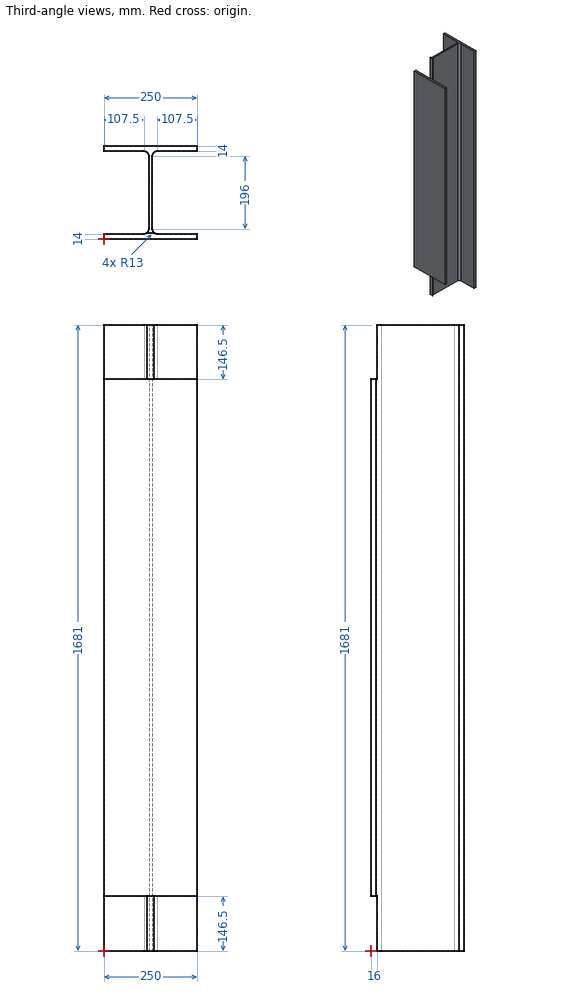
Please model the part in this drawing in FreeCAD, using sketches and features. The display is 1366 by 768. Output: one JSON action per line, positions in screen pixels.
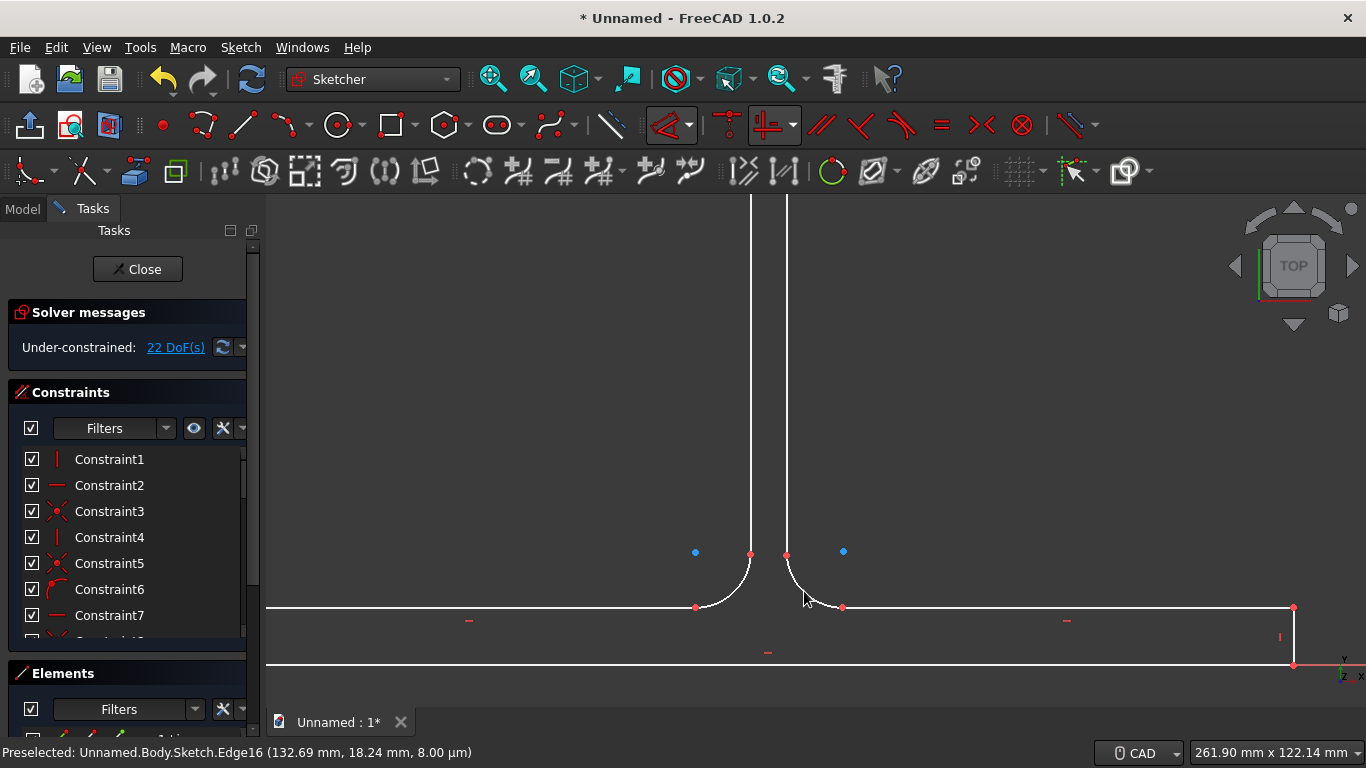
{"action": "left_click", "coordinate": [787, 309]}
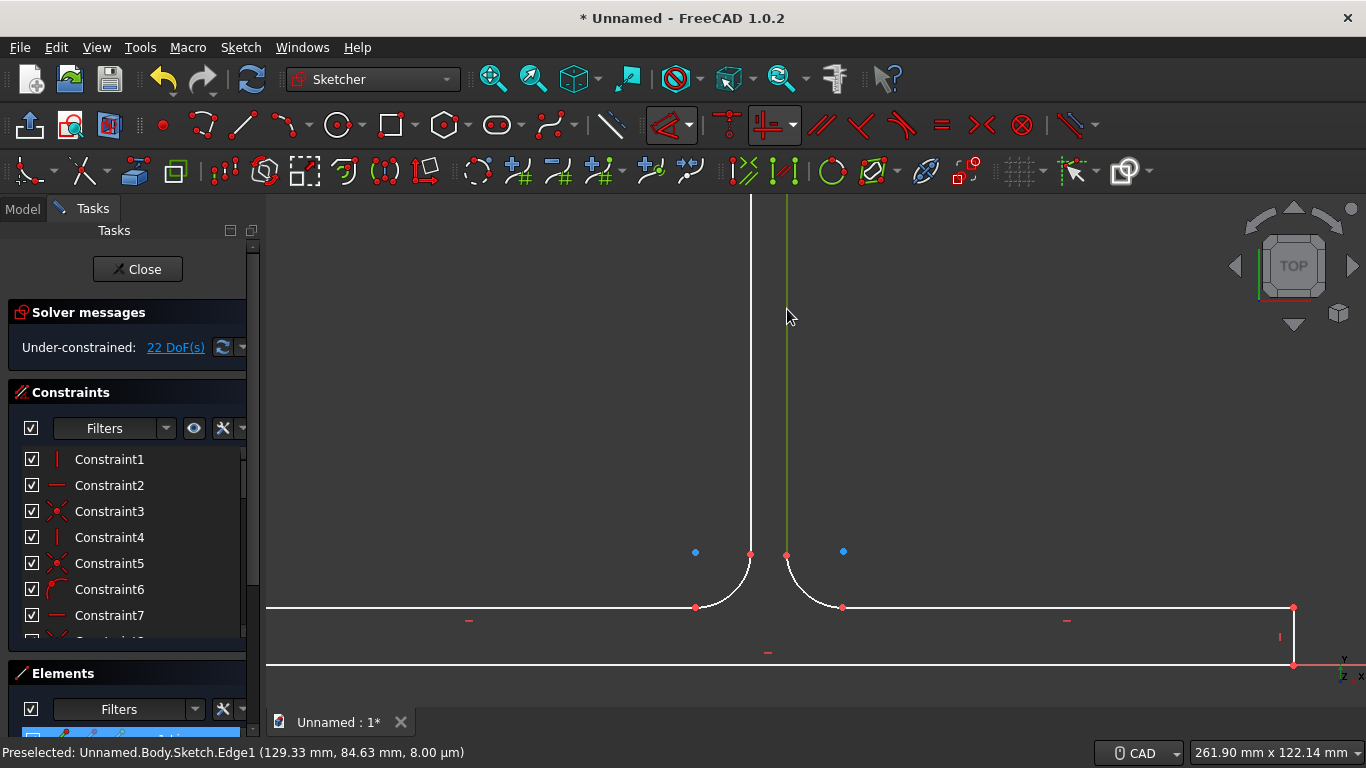
{"action": "scroll", "coordinate": [738, 584], "scroll_direction": "down", "scroll_amount": 6}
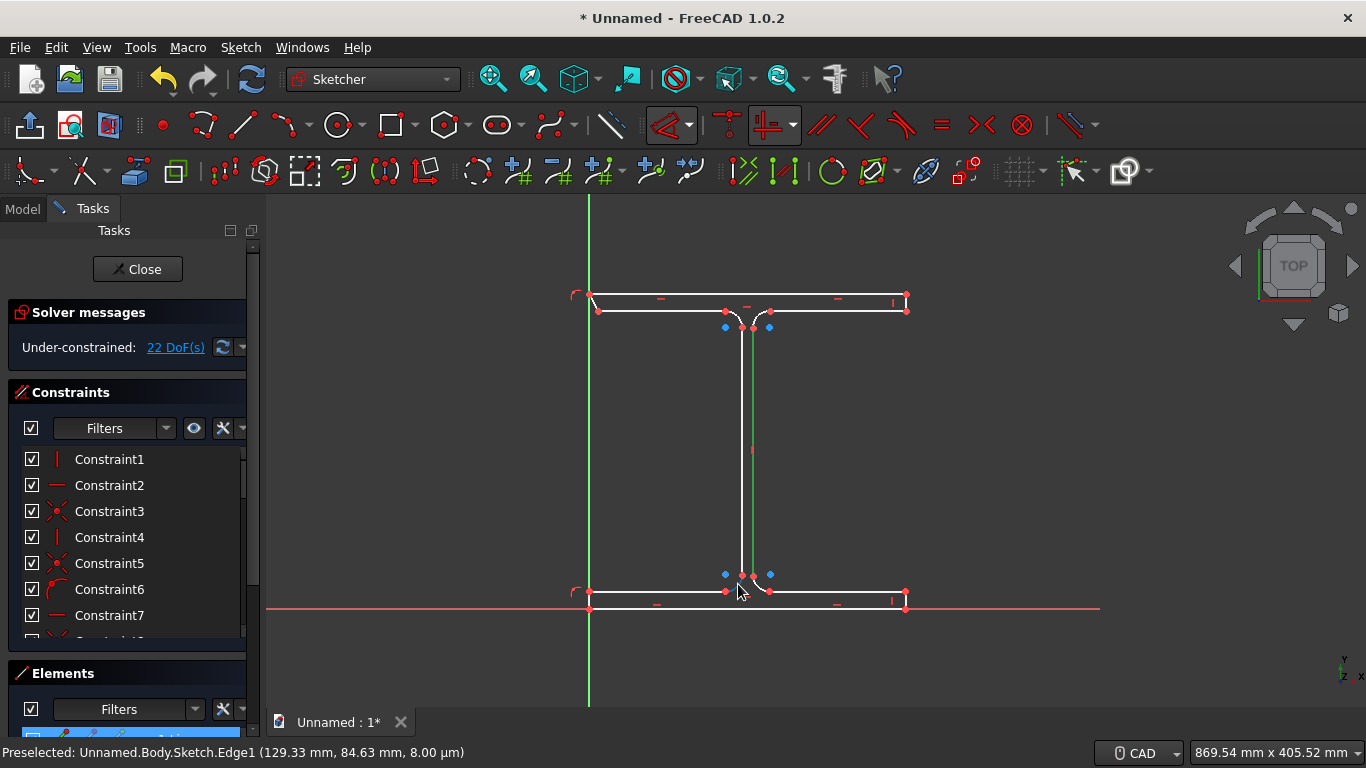
{"action": "scroll", "coordinate": [762, 313], "scroll_direction": "up", "scroll_amount": 3}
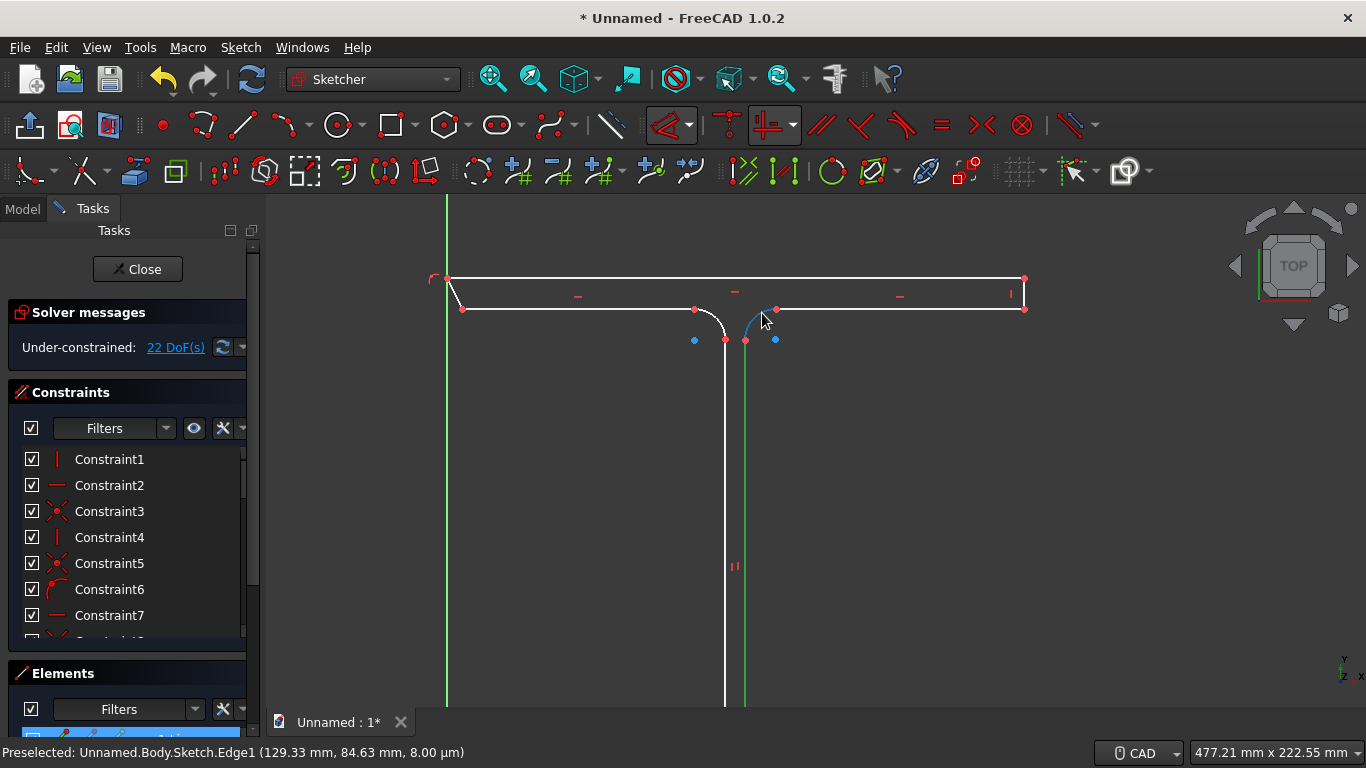
{"action": "left_click", "coordinate": [762, 312]}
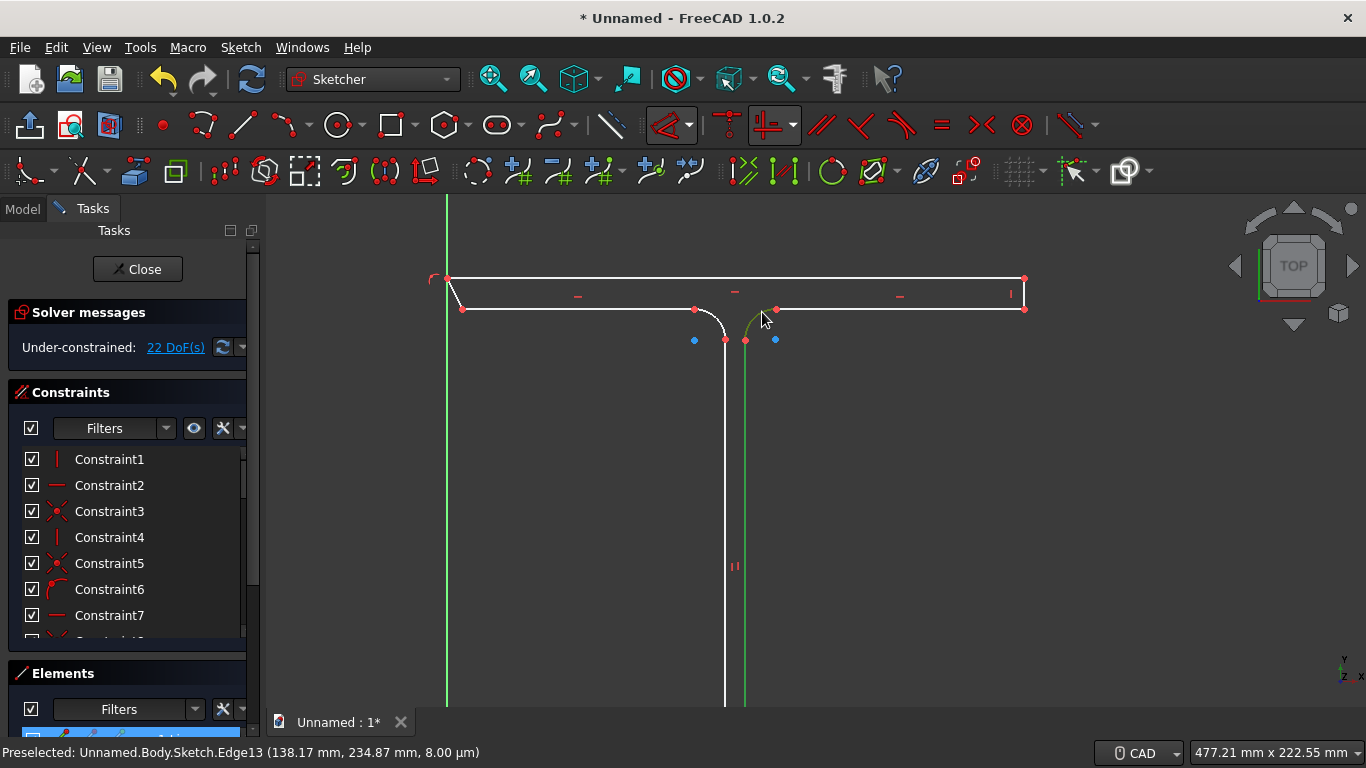
{"action": "left_click", "coordinate": [902, 126]}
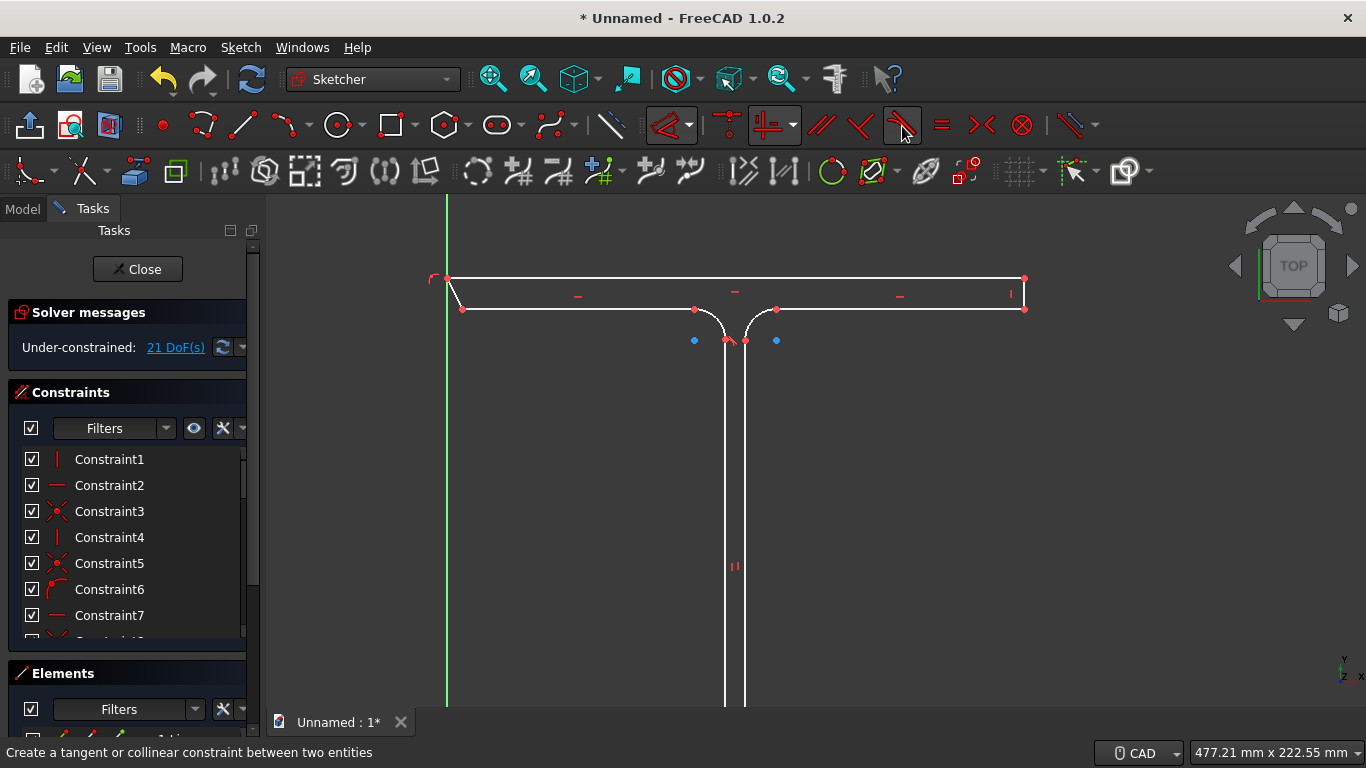
{"action": "left_click", "coordinate": [745, 657]}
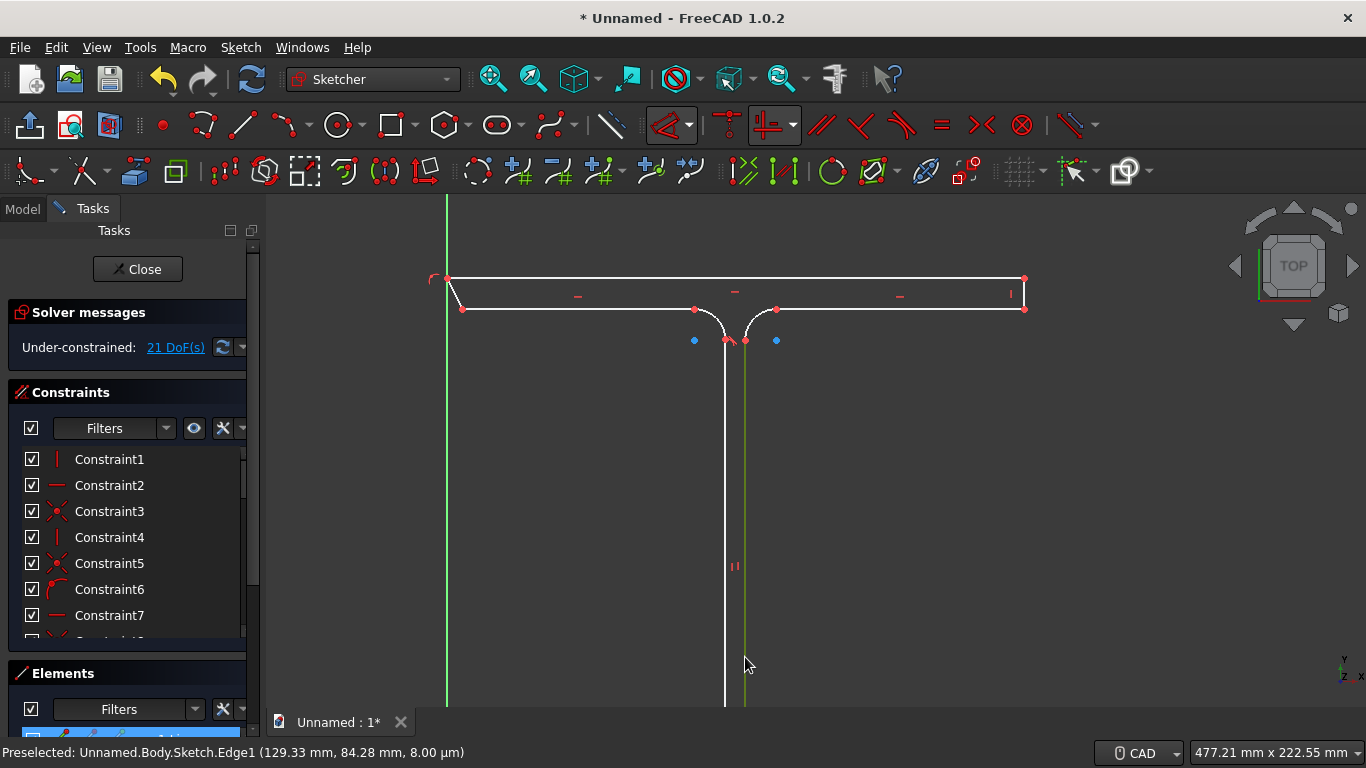
{"action": "scroll", "coordinate": [762, 312], "scroll_direction": "down", "scroll_amount": 3}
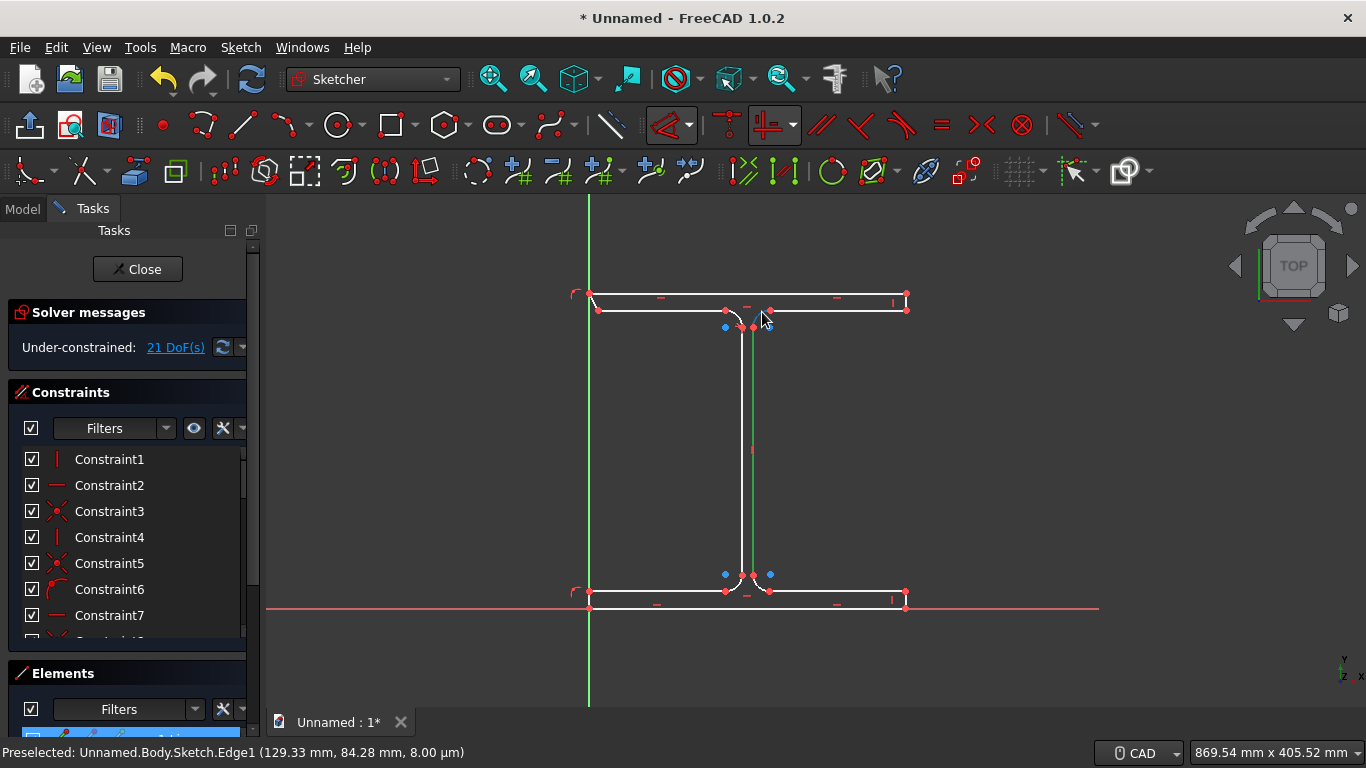
{"action": "scroll", "coordinate": [755, 583], "scroll_direction": "up", "scroll_amount": 4}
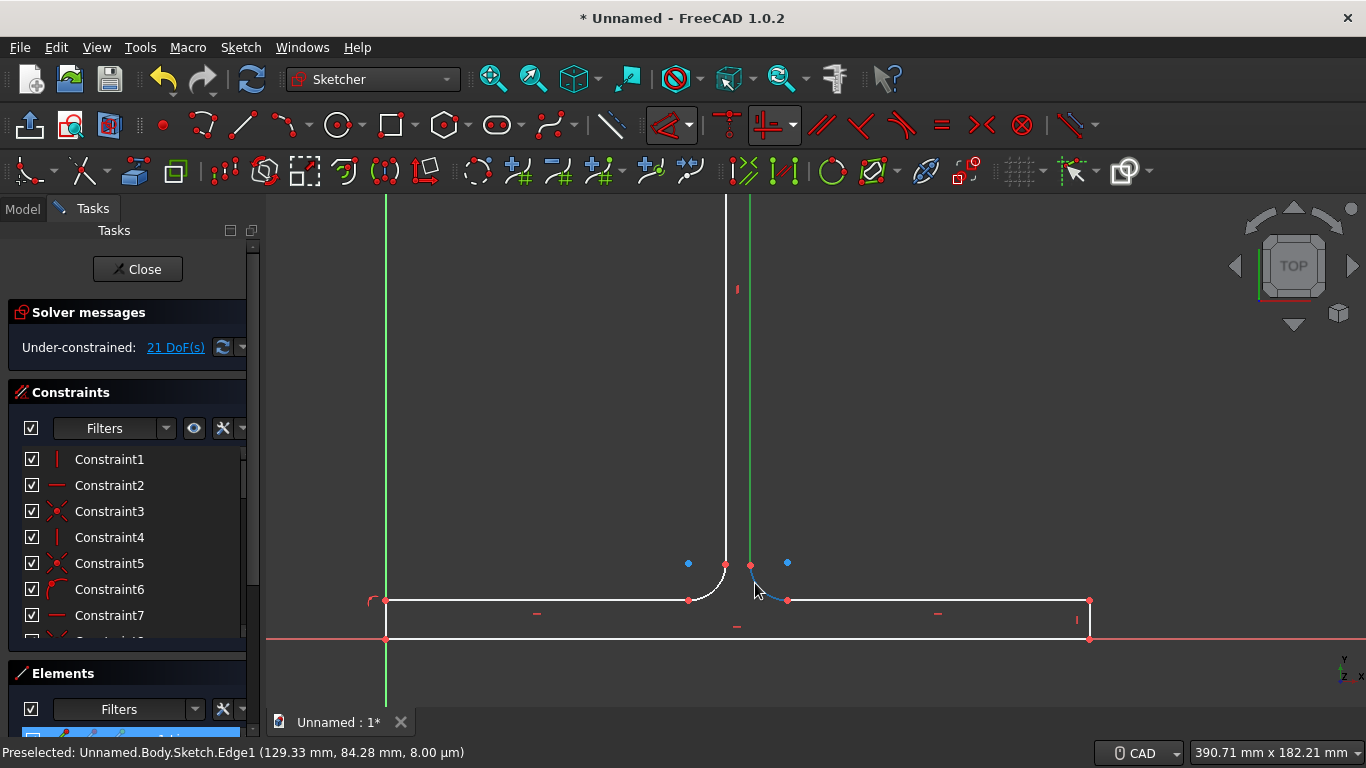
{"action": "left_click", "coordinate": [755, 581]}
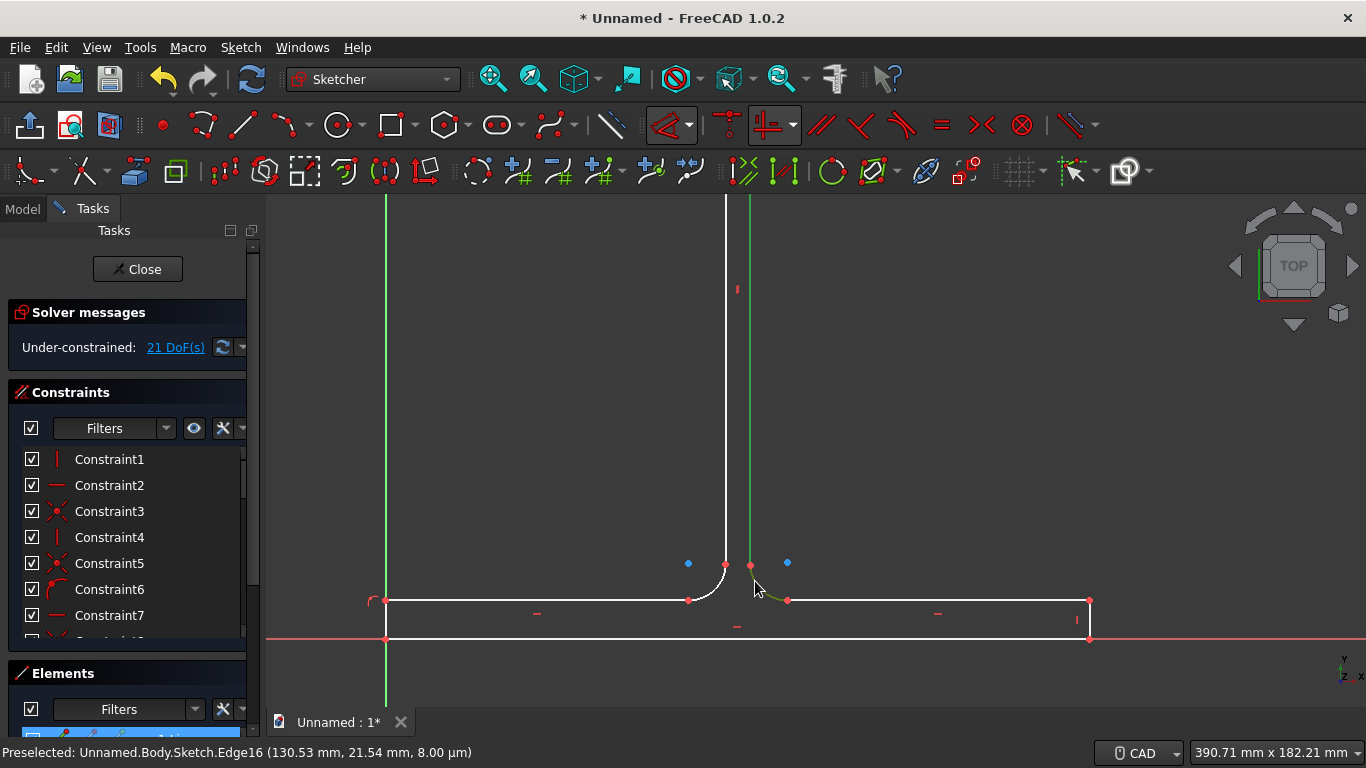
{"action": "left_click", "coordinate": [902, 126]}